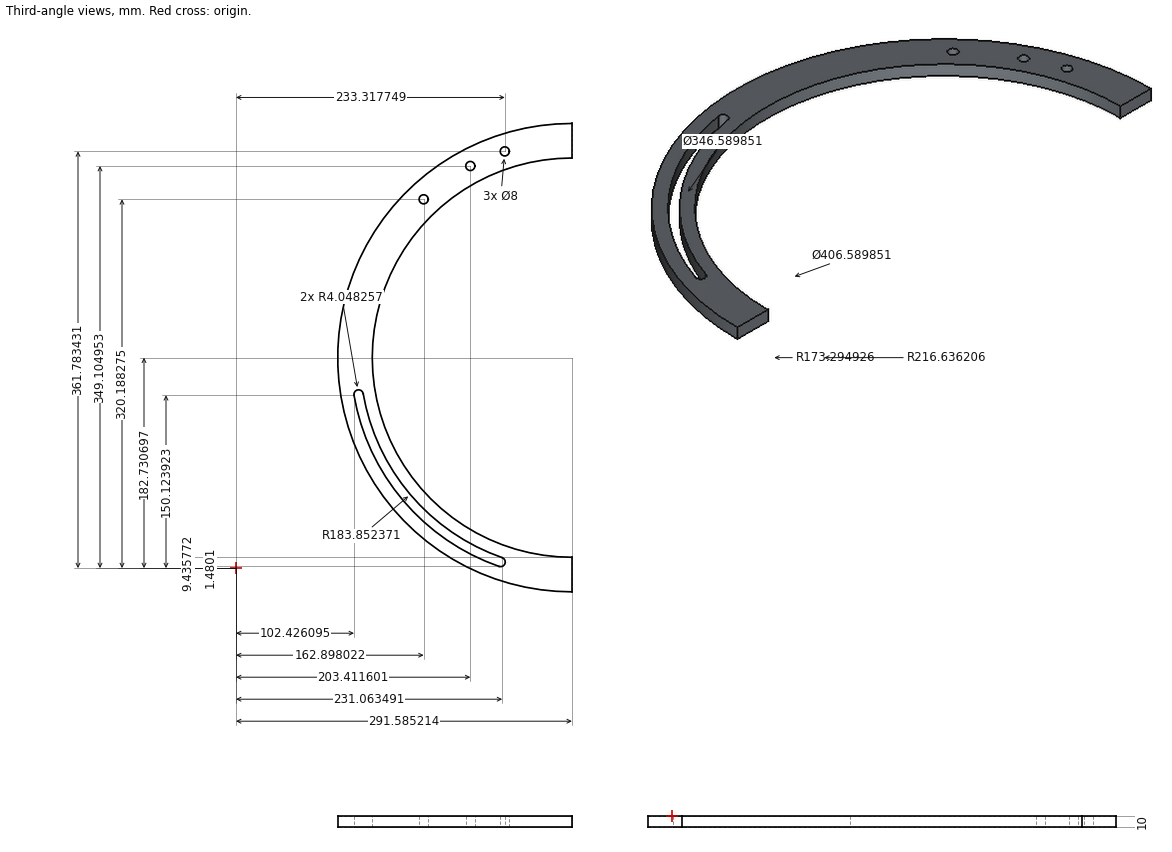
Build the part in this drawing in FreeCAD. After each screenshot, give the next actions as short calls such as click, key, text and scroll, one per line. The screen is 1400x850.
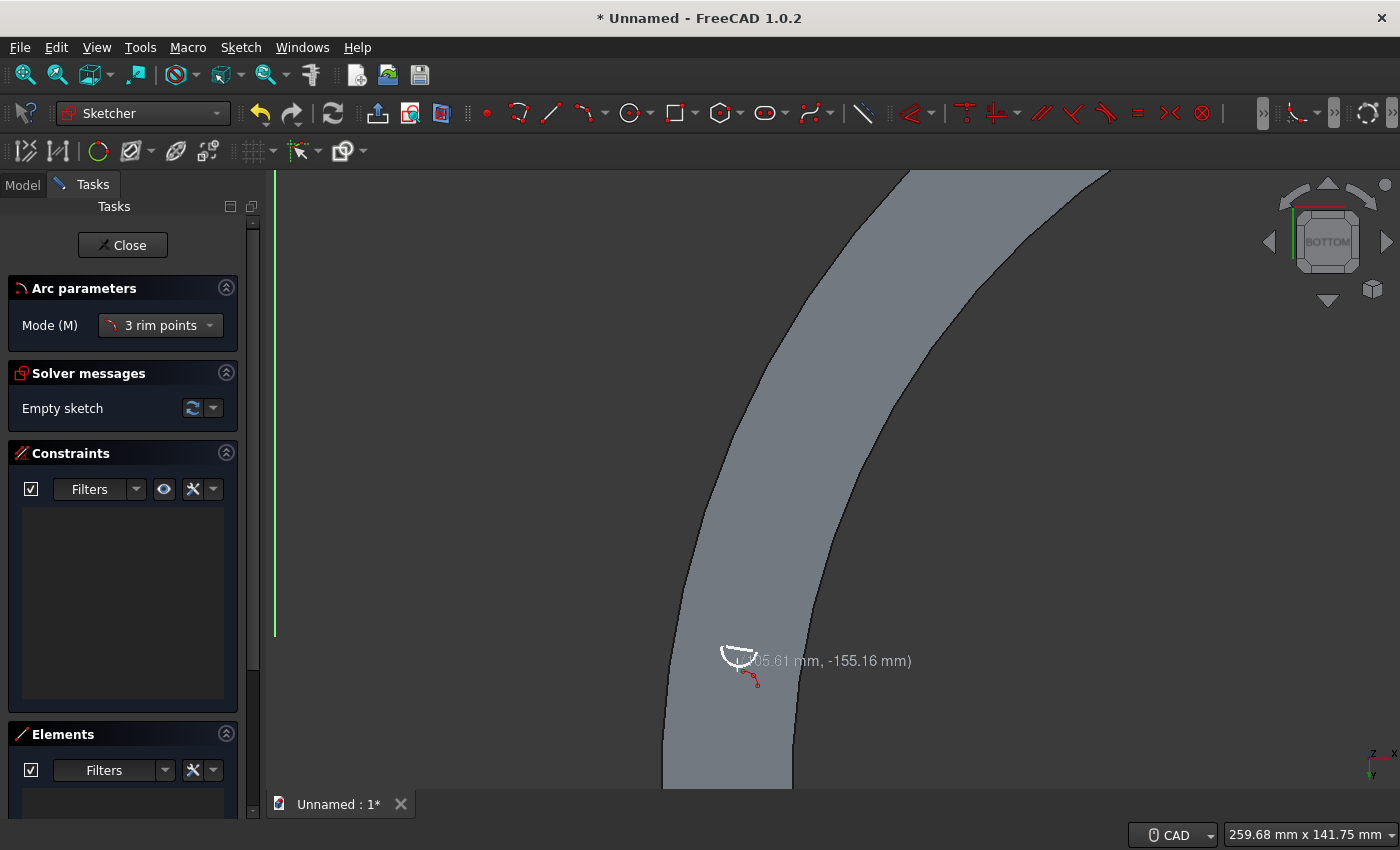
click(737, 665)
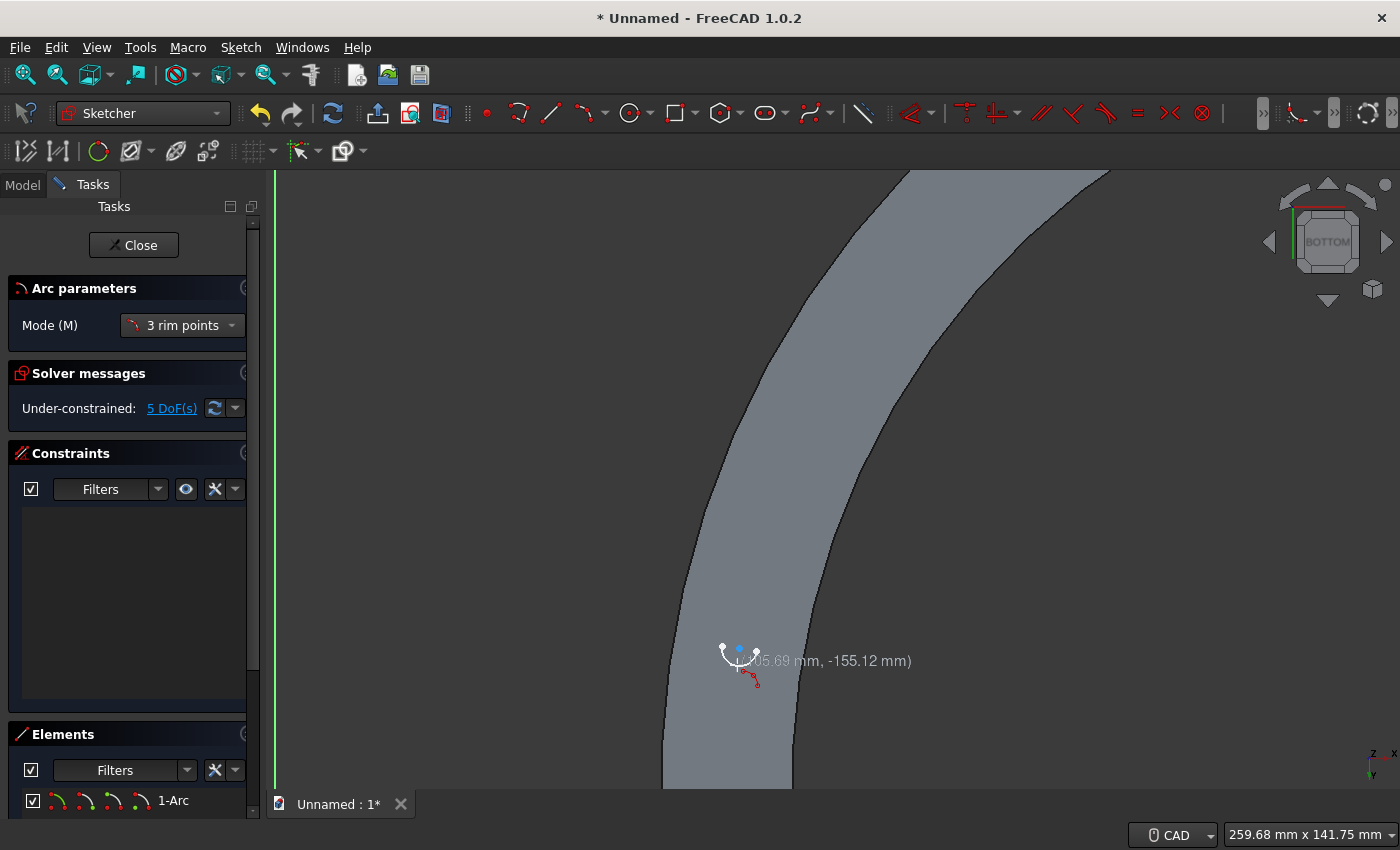
click(757, 652)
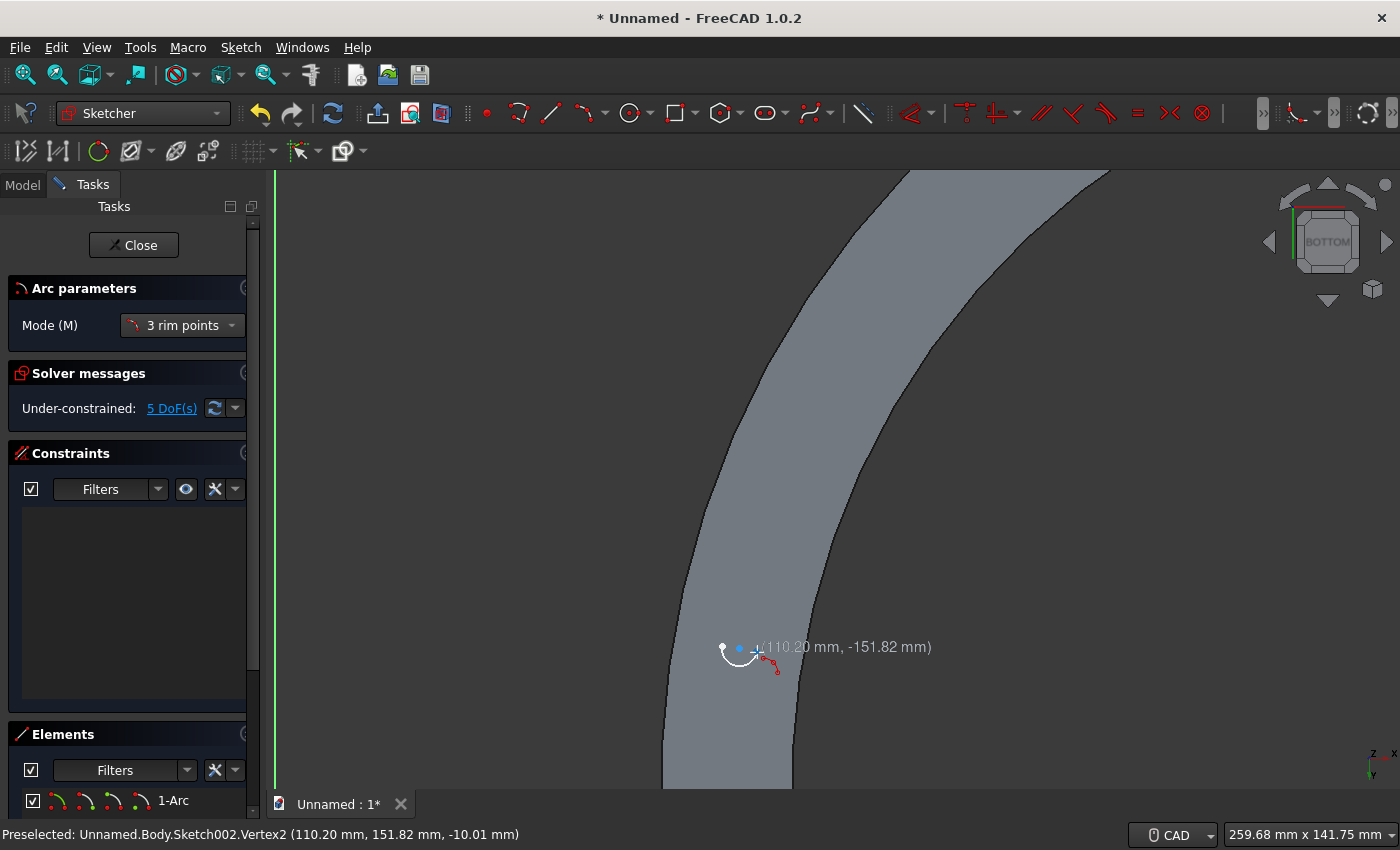
scroll(739, 665, down, 3)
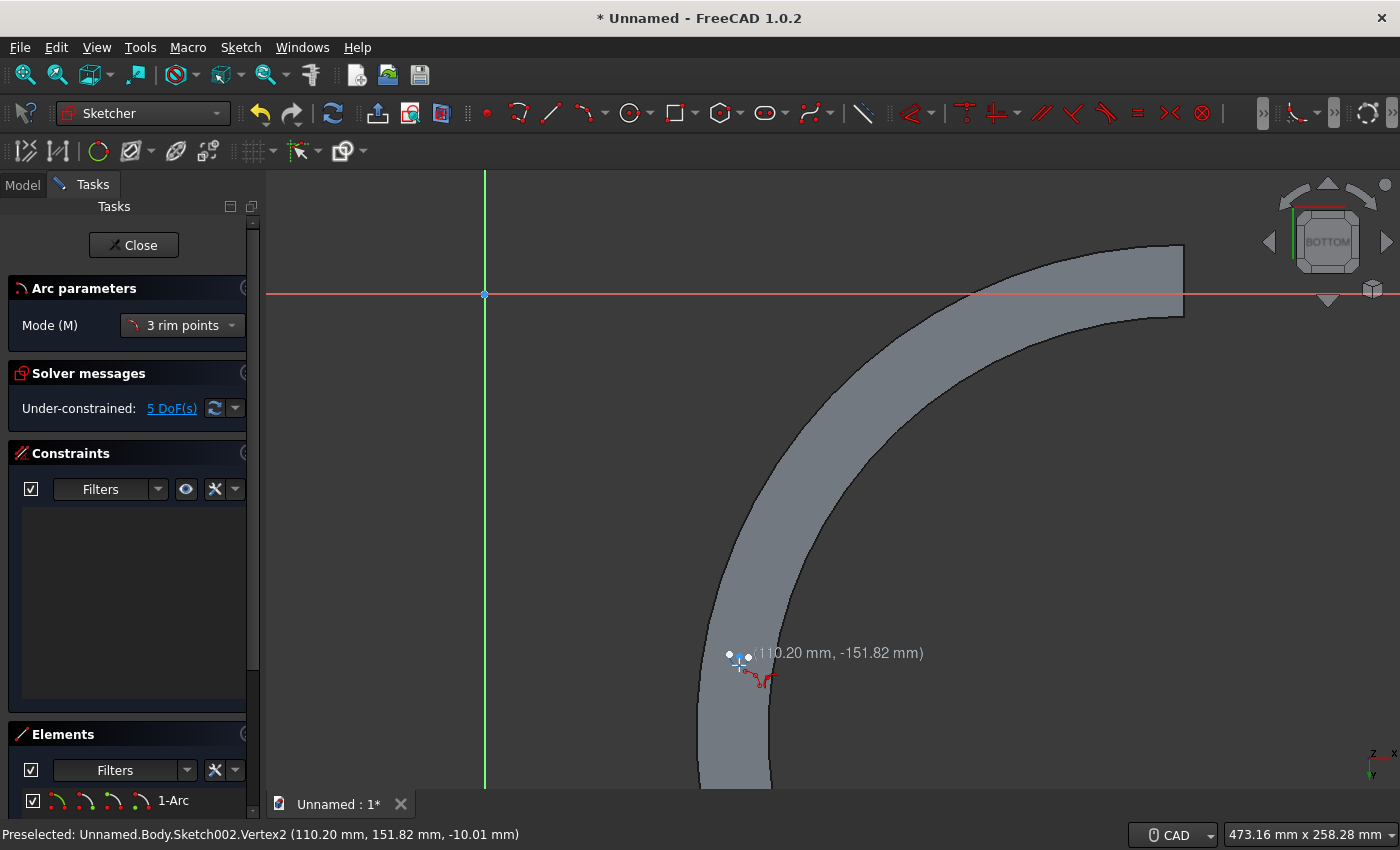
click(1039, 316)
click(847, 447)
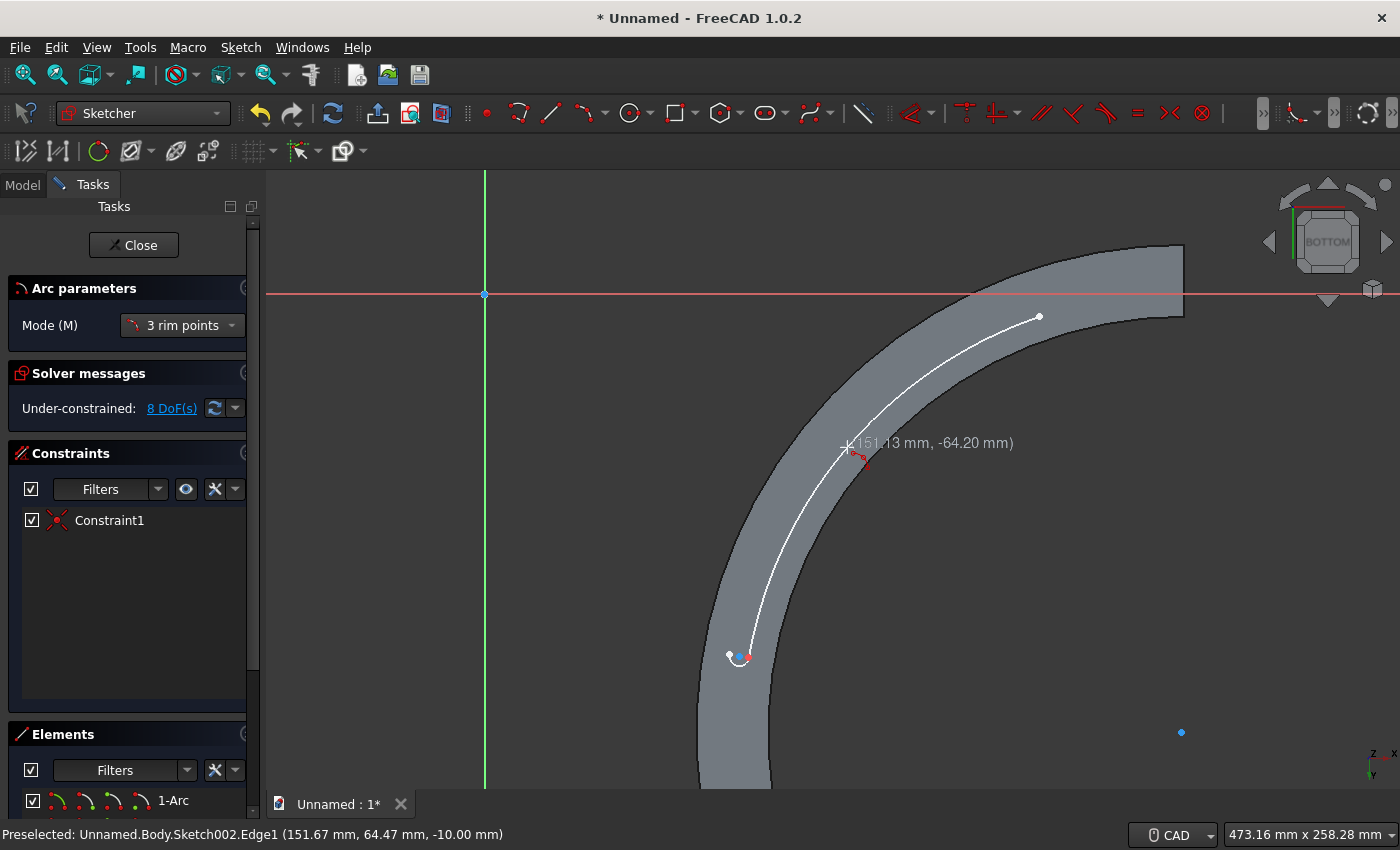
click(1039, 317)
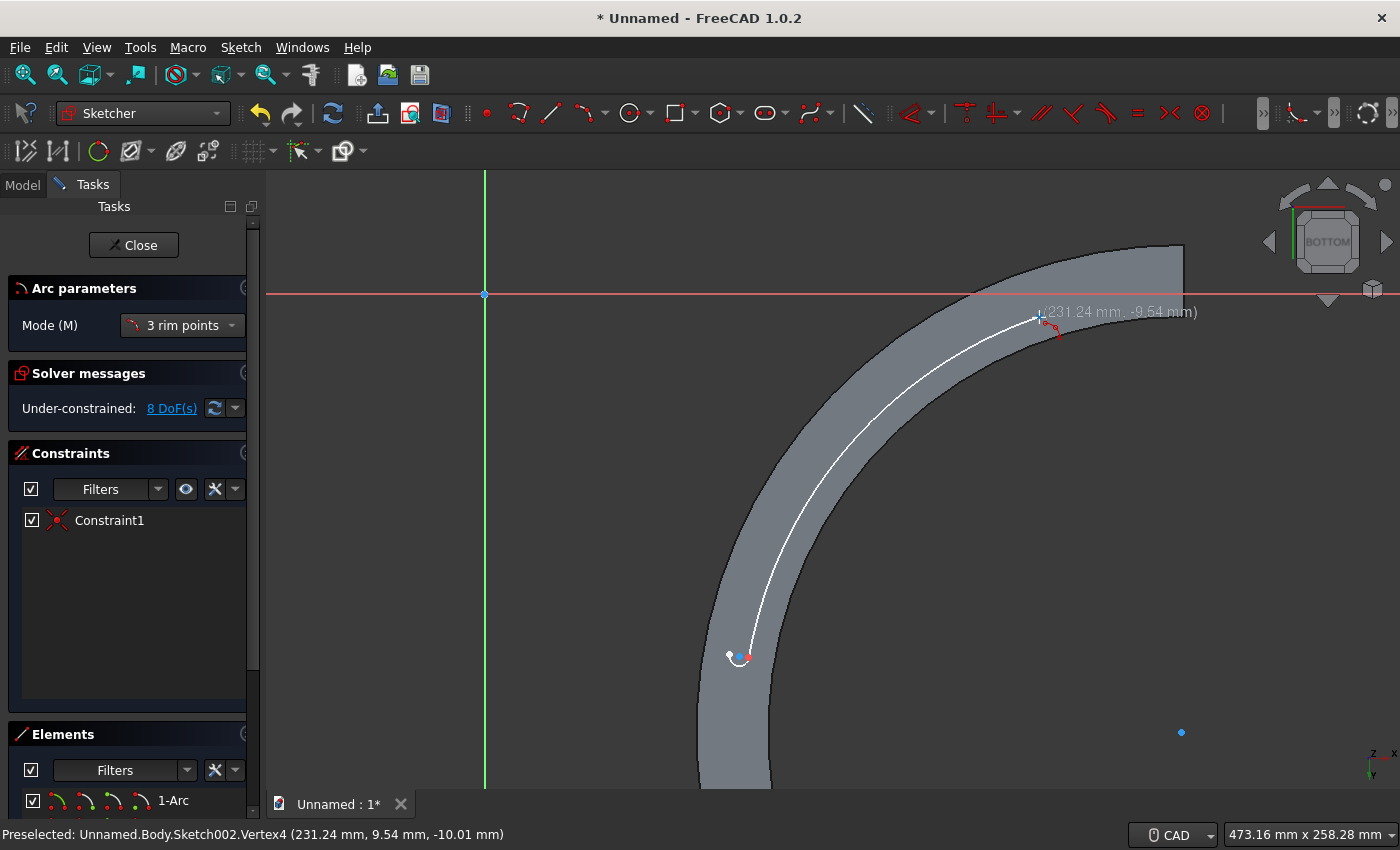
scroll(1032, 298, up, 8)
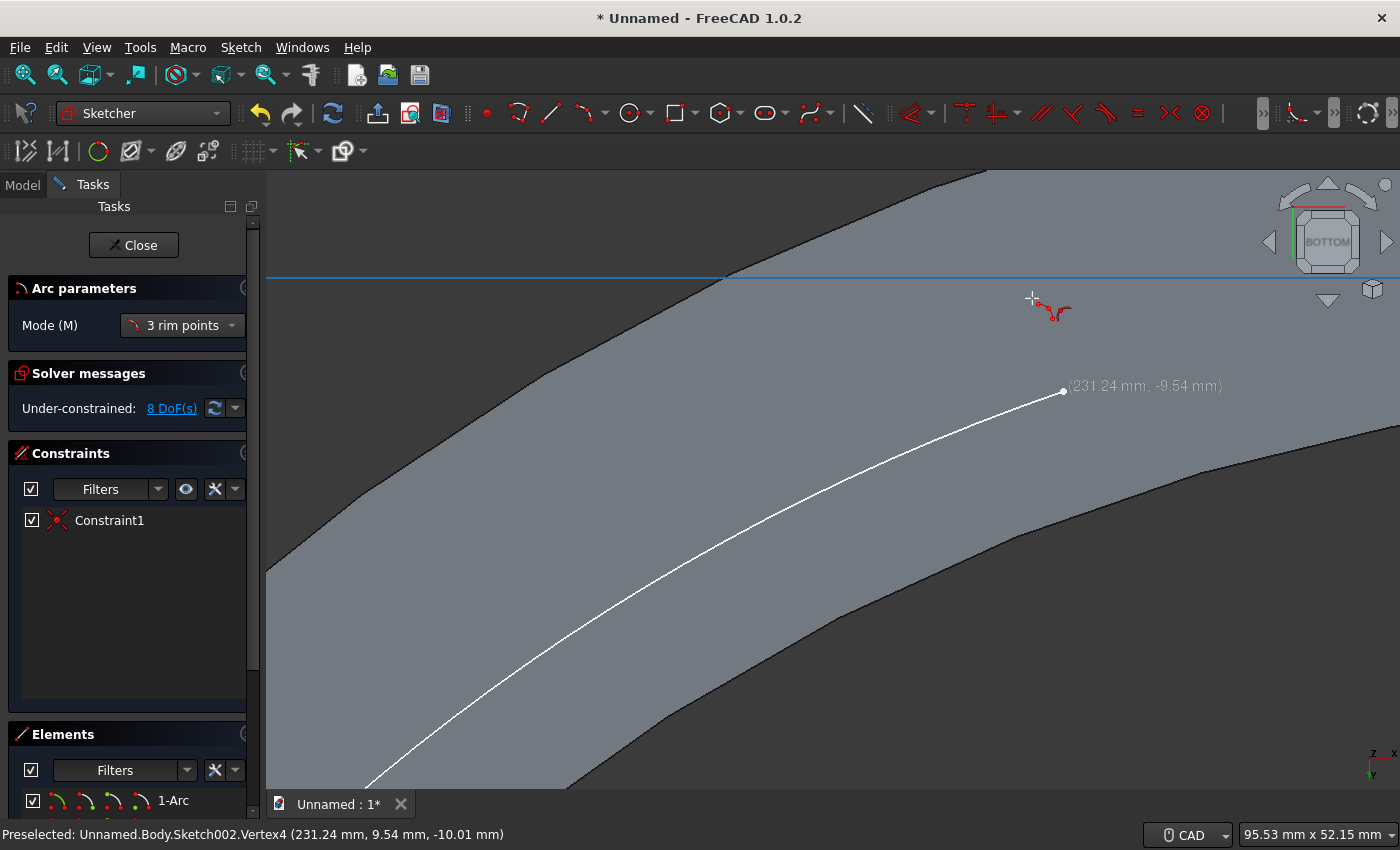
click(1030, 296)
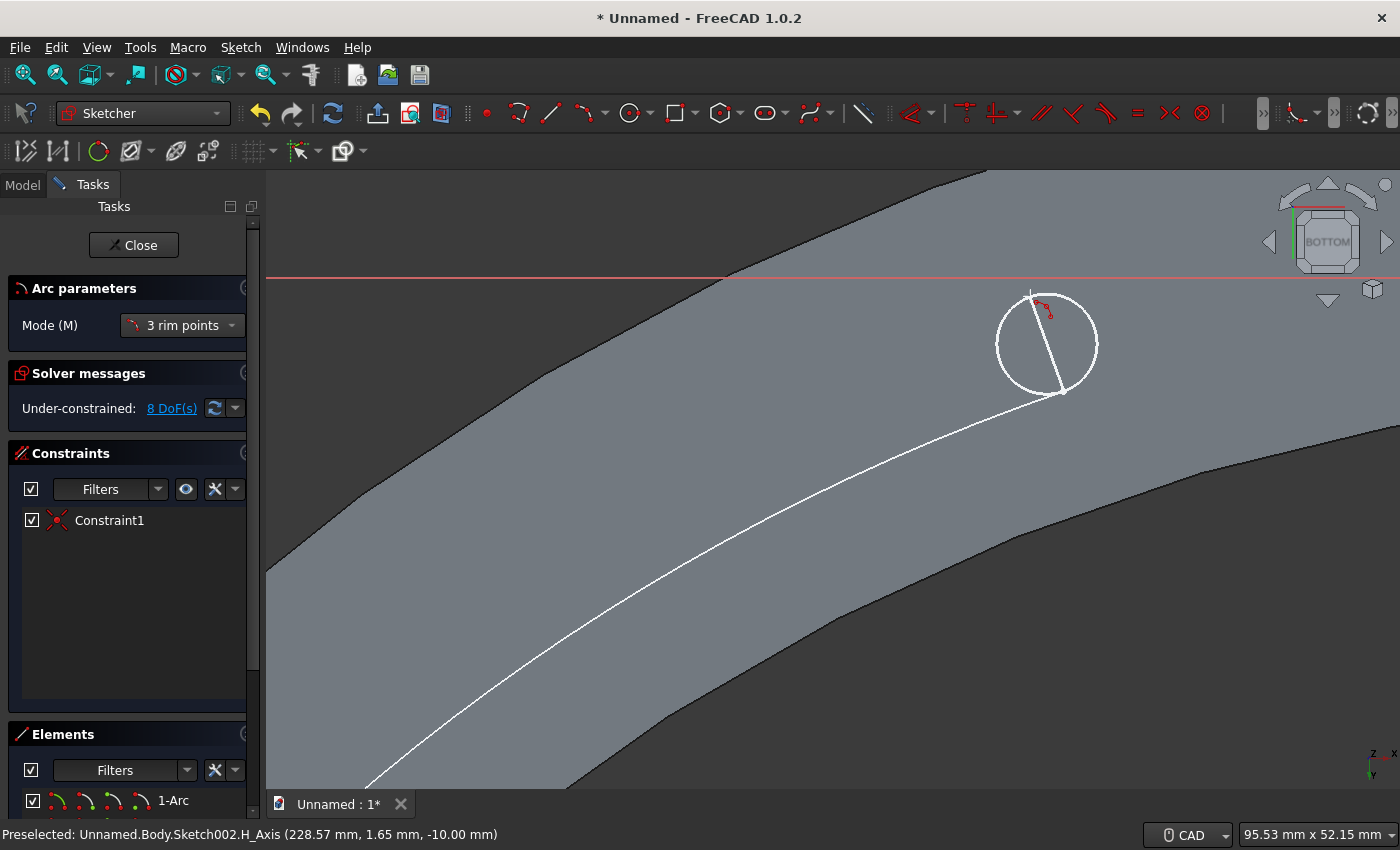
scroll(1032, 298, down, 8)